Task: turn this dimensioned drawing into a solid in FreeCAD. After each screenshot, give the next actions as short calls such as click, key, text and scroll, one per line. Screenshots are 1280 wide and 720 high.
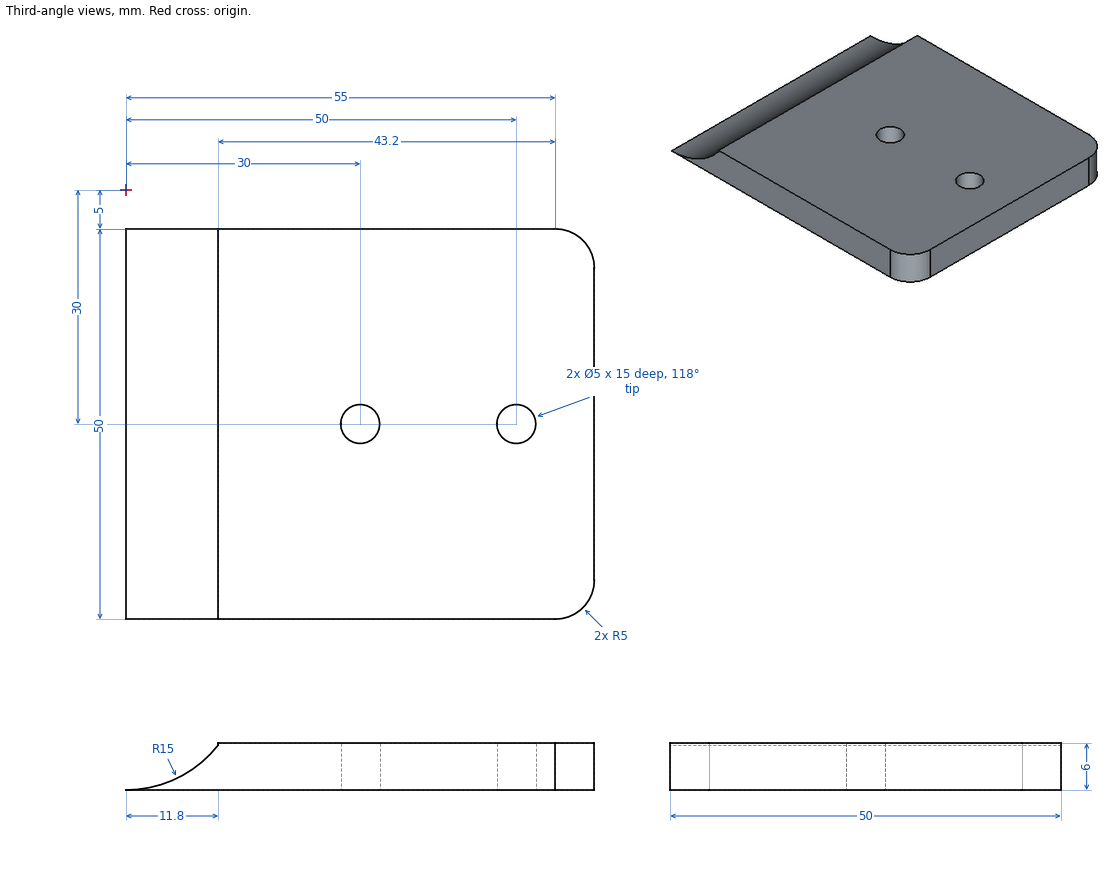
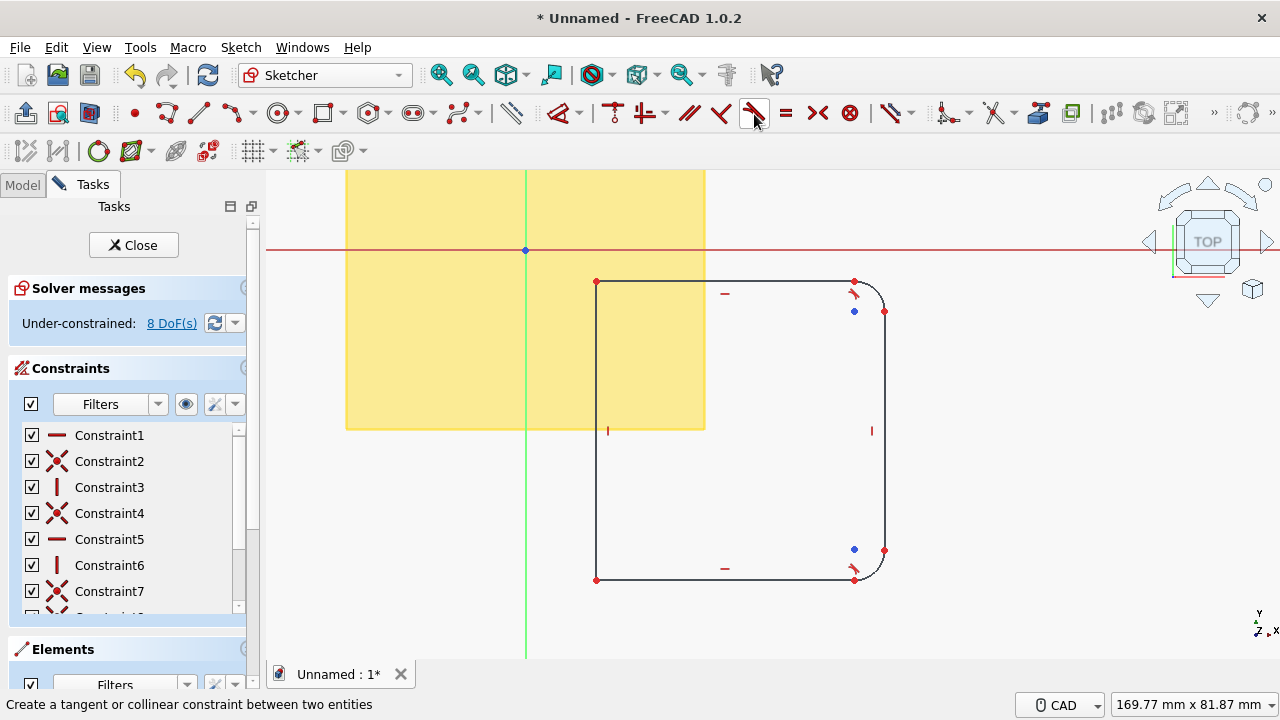
click(885, 479)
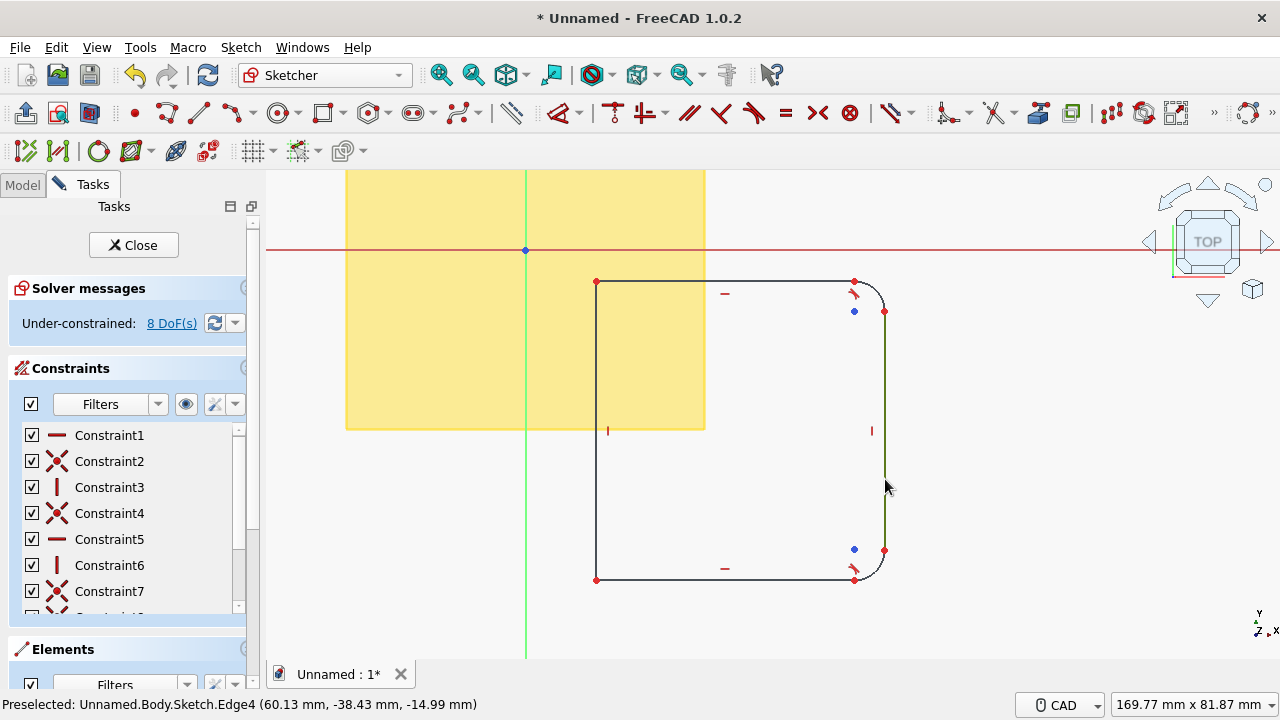
click(868, 577)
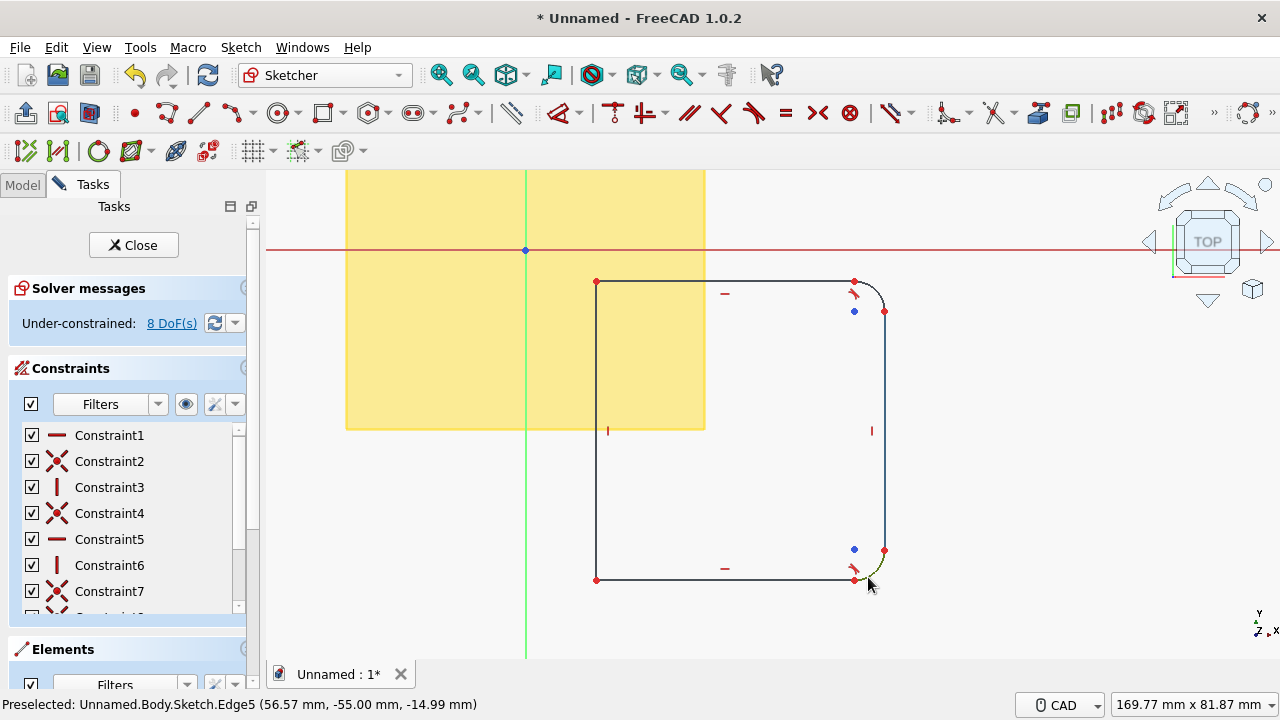
click(754, 114)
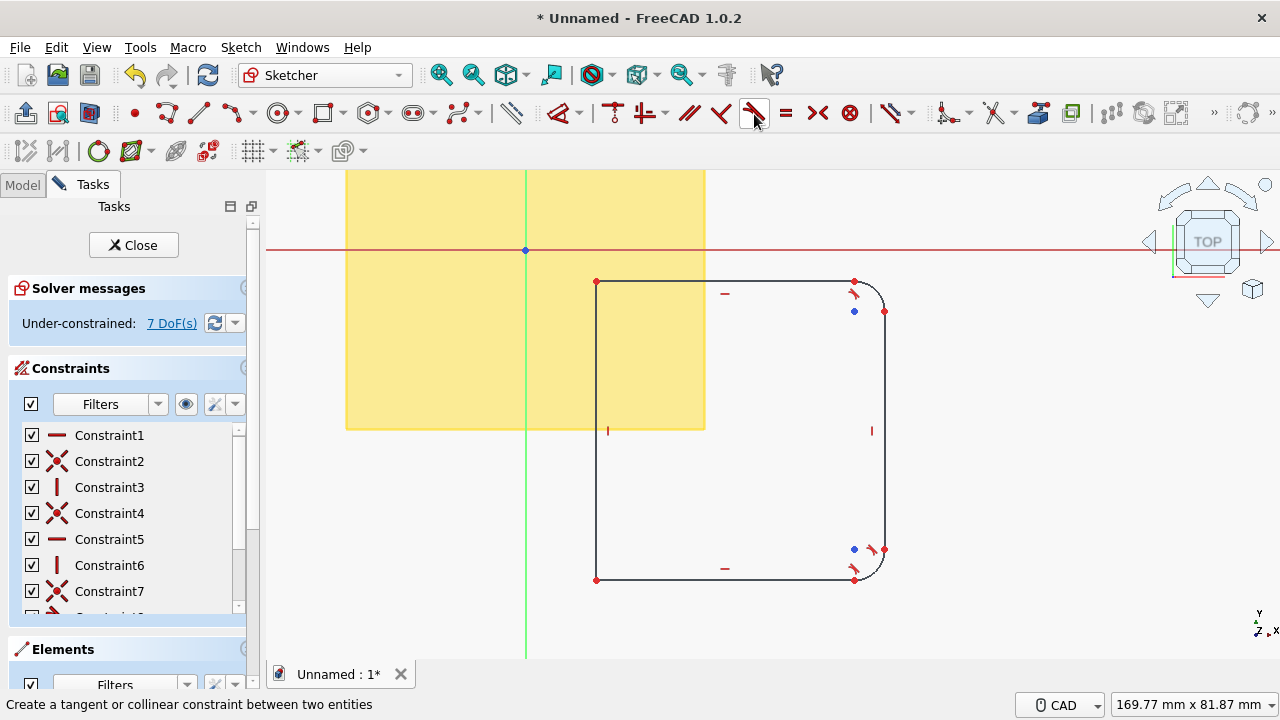
click(885, 478)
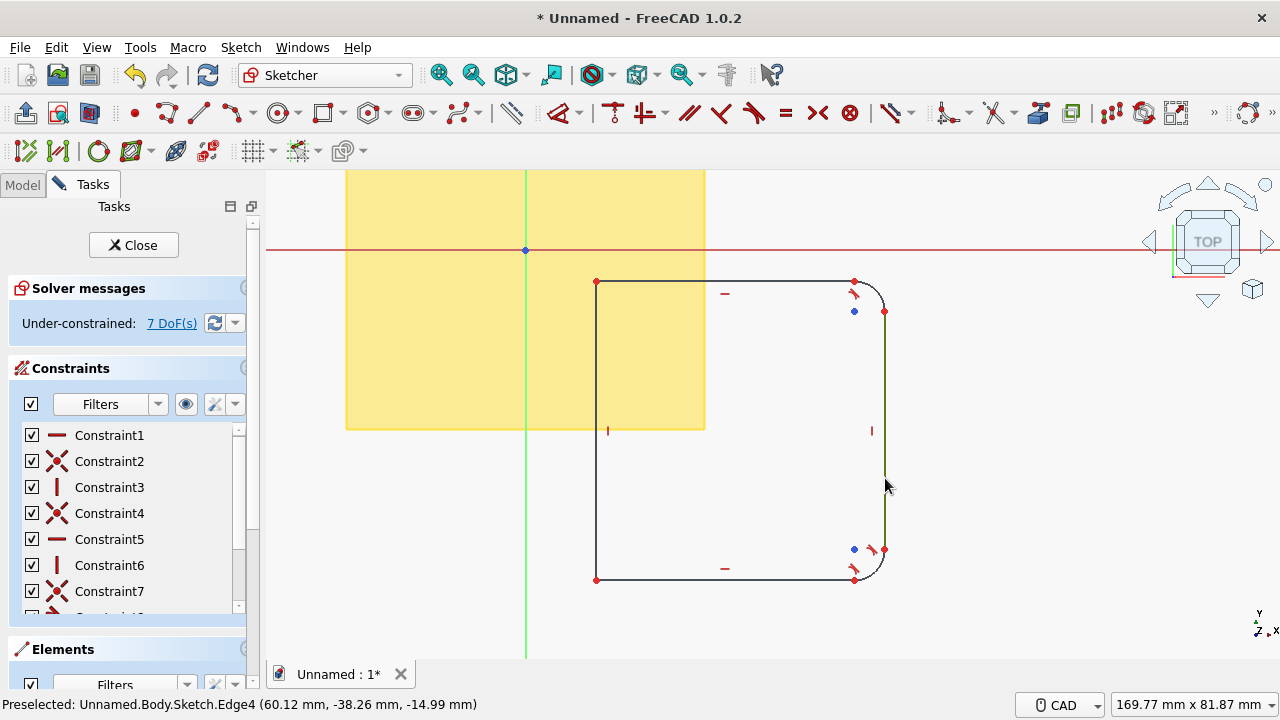
click(881, 298)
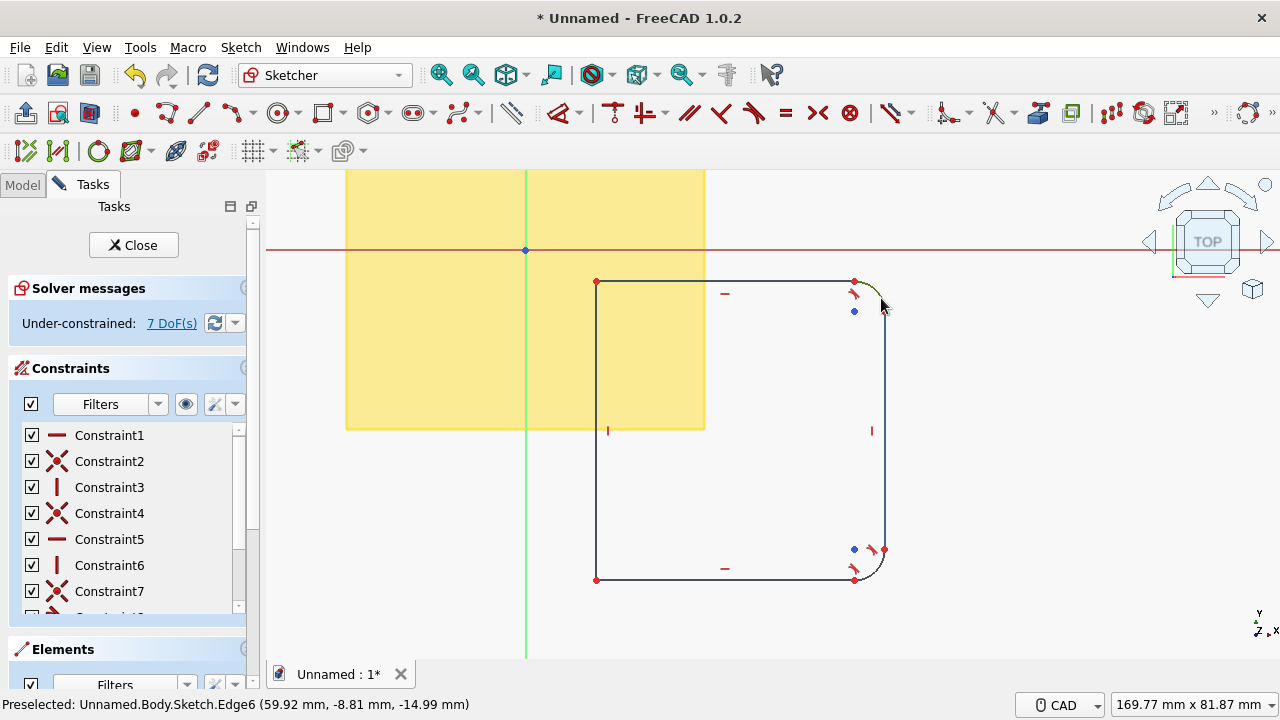
click(754, 114)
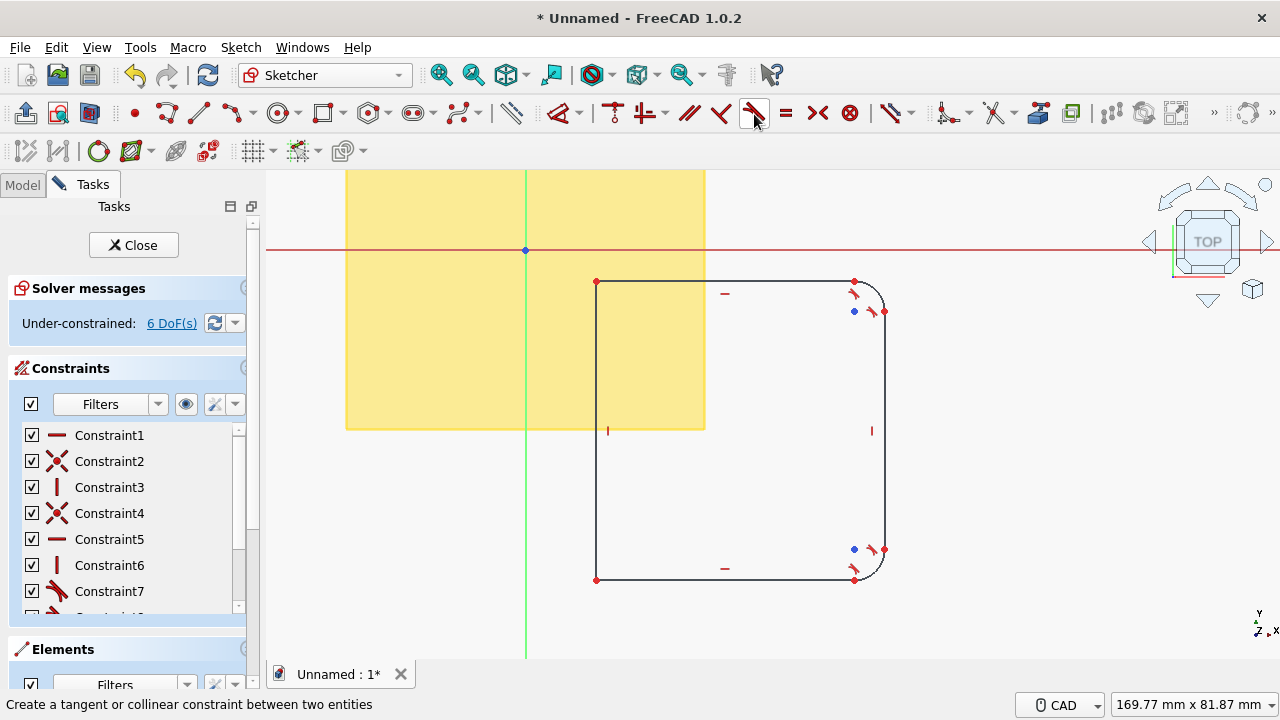
click(868, 577)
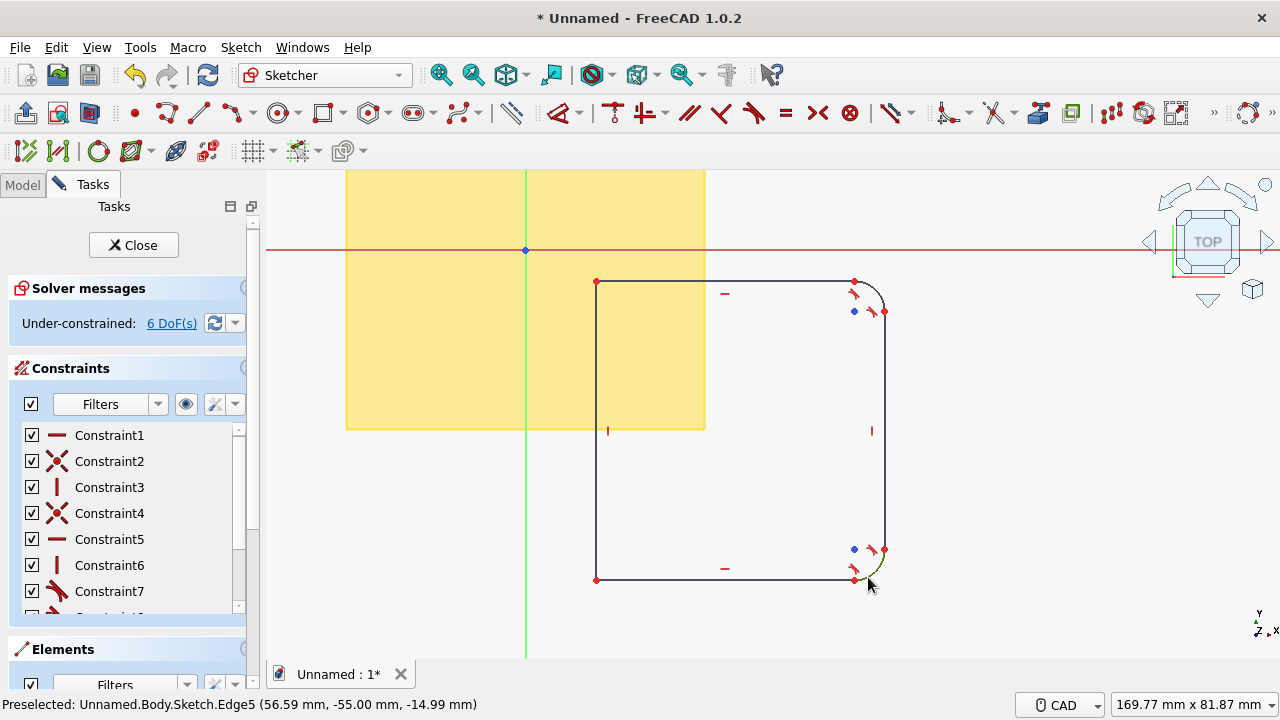
click(881, 298)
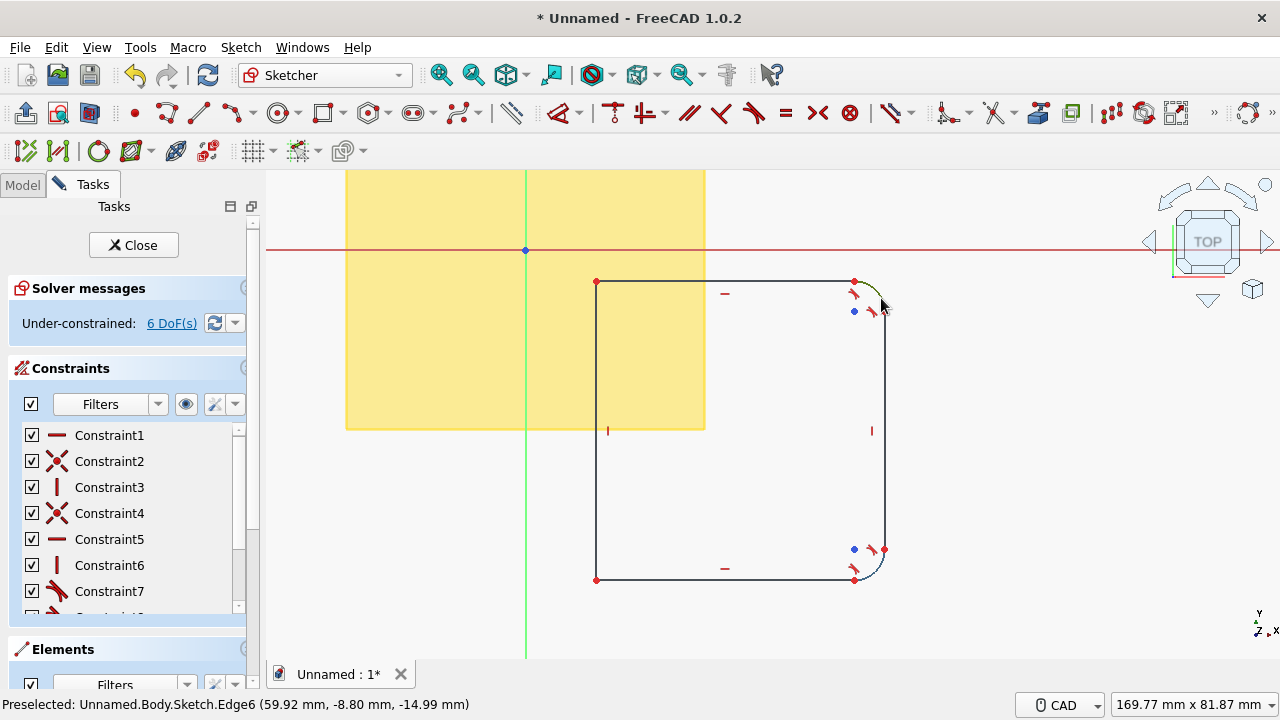
click(786, 114)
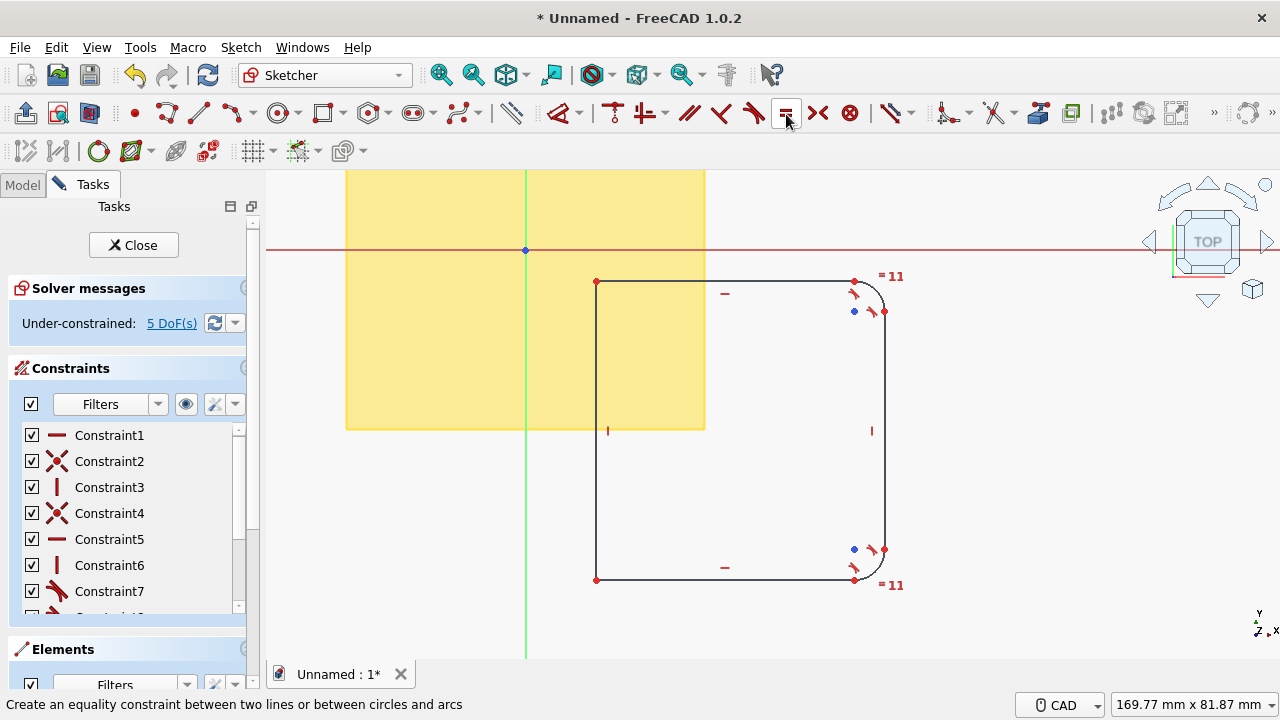
click(558, 114)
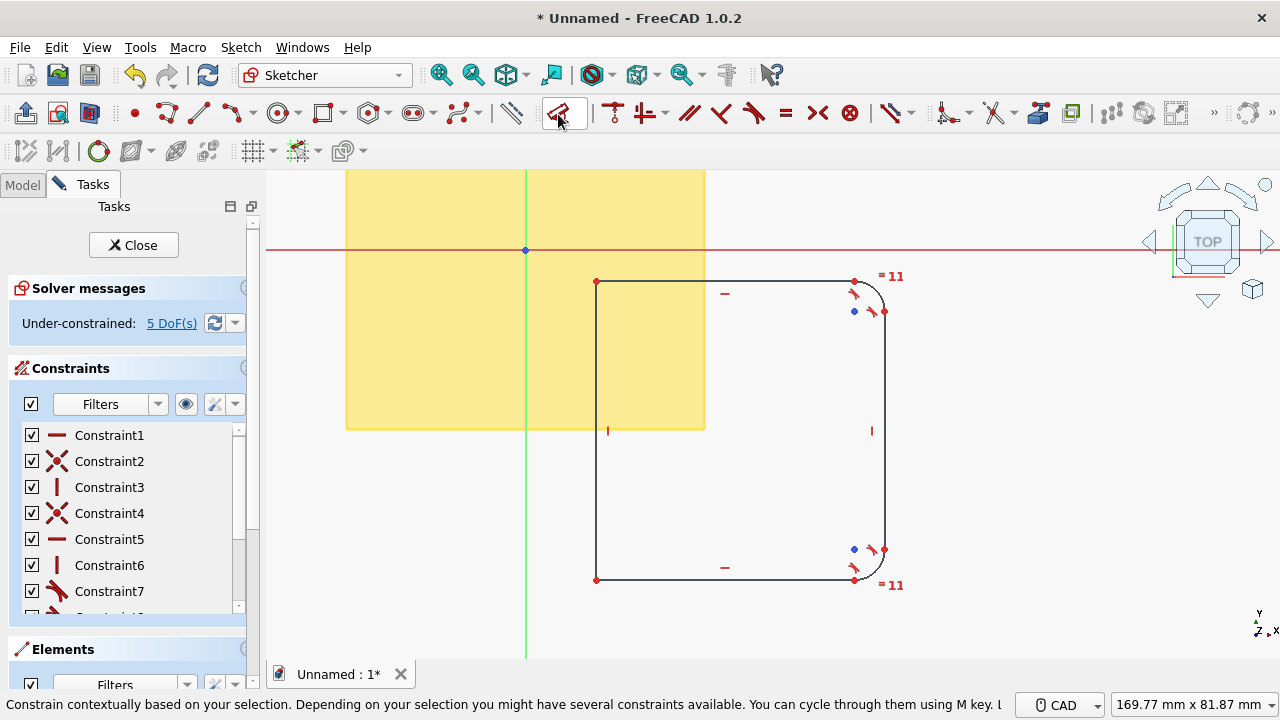
scroll(868, 577, up, 2)